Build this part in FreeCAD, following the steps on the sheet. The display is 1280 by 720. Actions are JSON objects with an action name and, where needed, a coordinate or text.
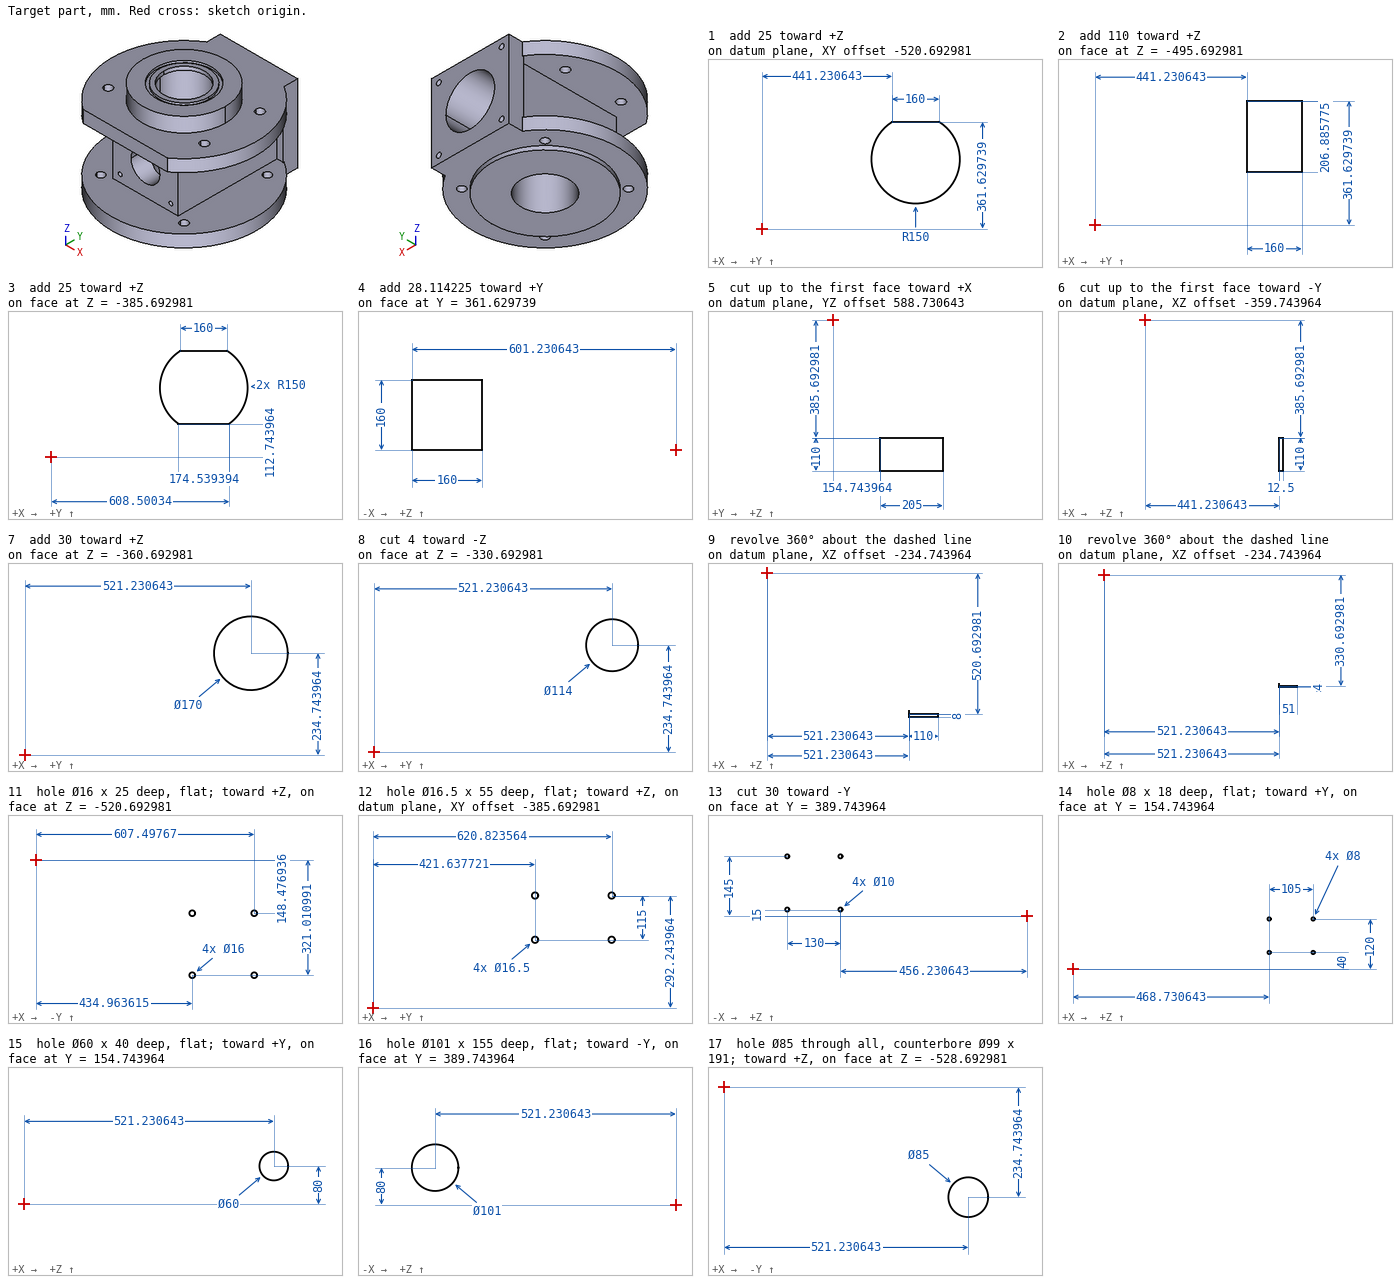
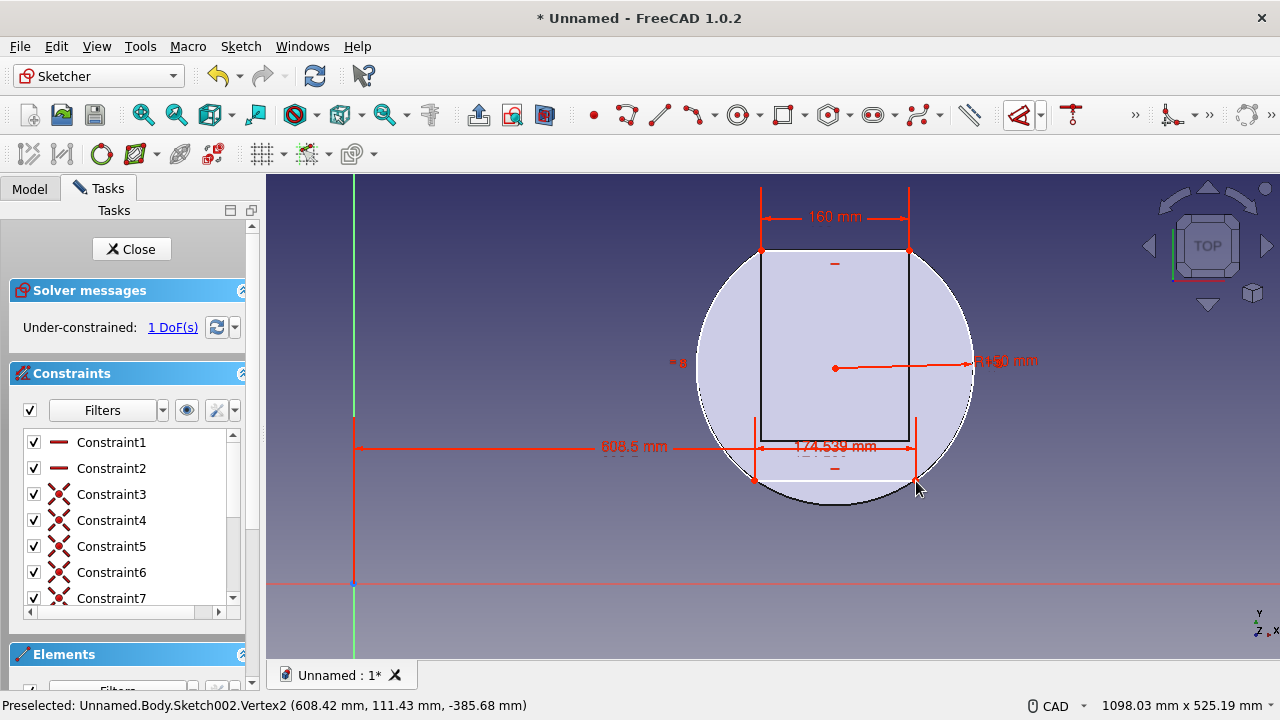
{"action": "left_click", "coordinate": [755, 481]}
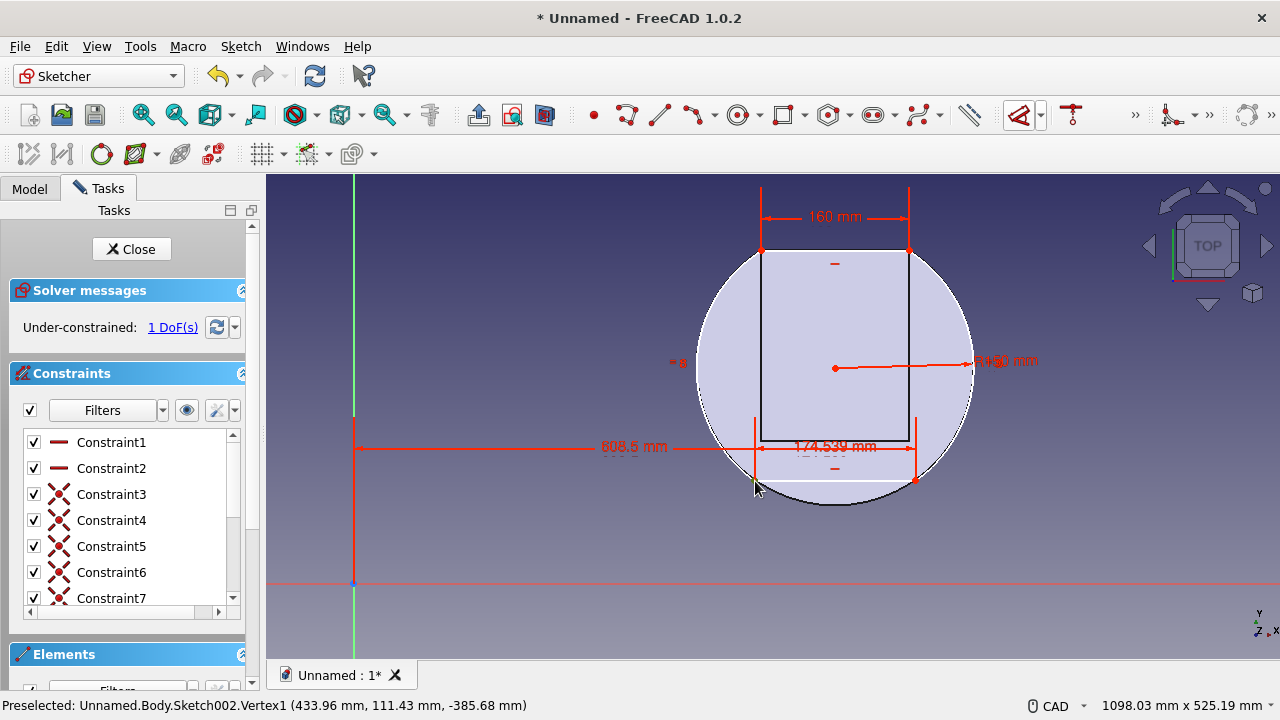
{"action": "left_click", "coordinate": [1040, 116]}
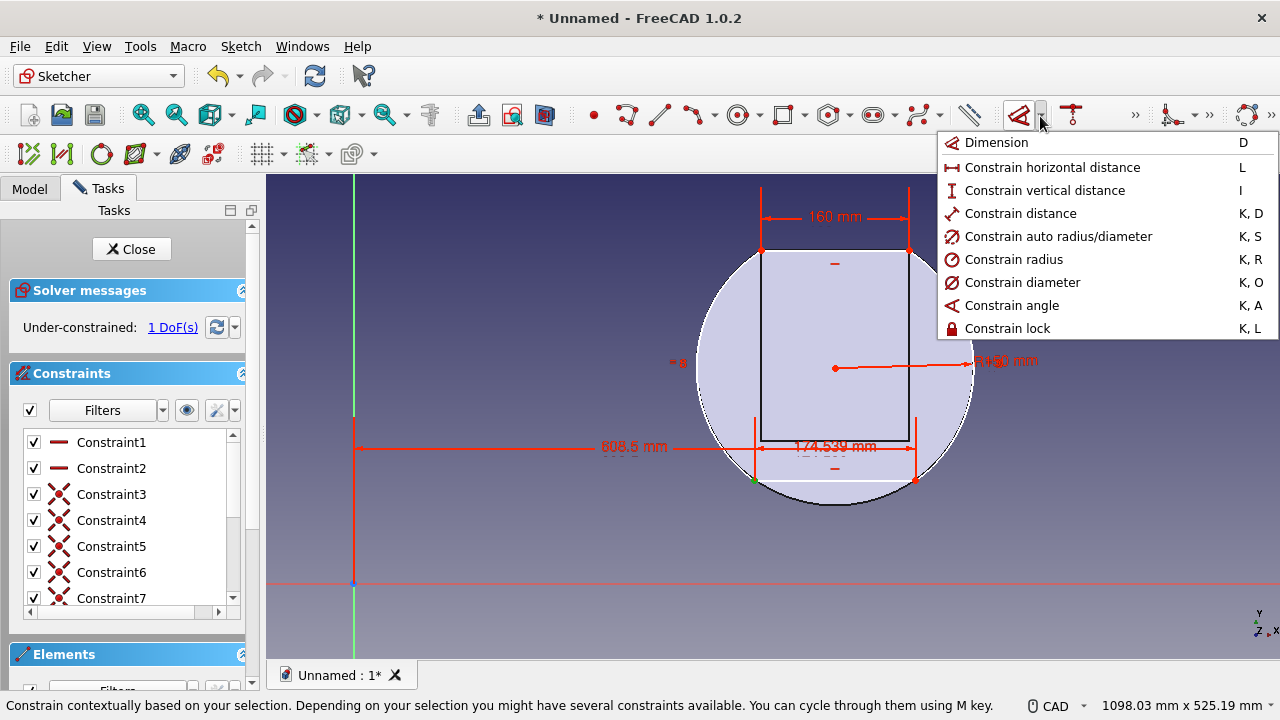
{"action": "left_click", "coordinate": [1108, 190]}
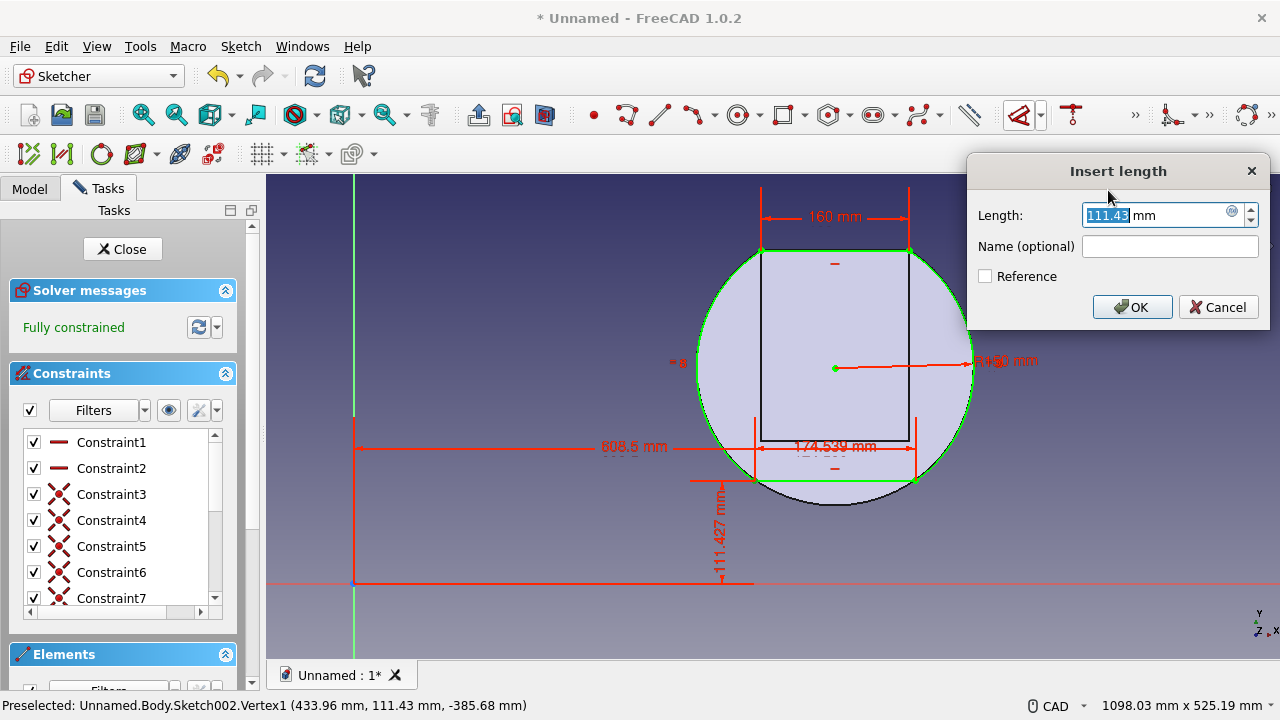
{"action": "type", "text": "112.743964"}
{"action": "key", "text": "Return"}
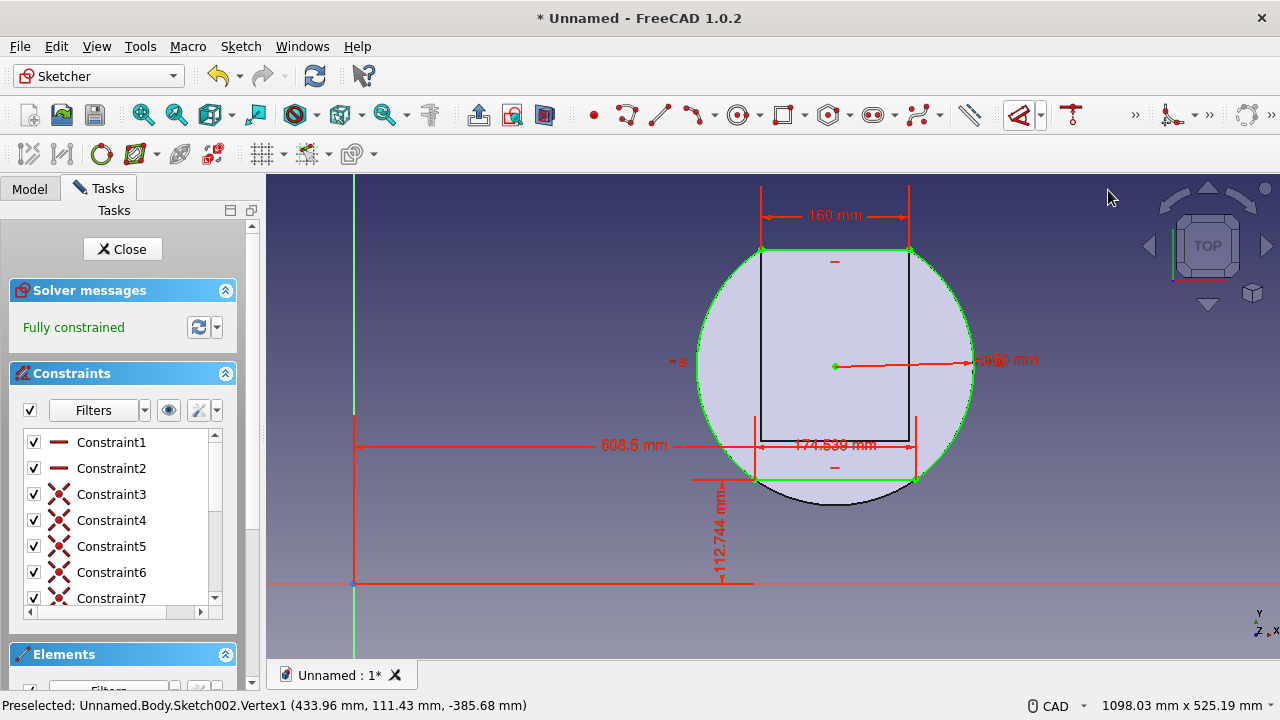
{"action": "left_click", "coordinate": [123, 249]}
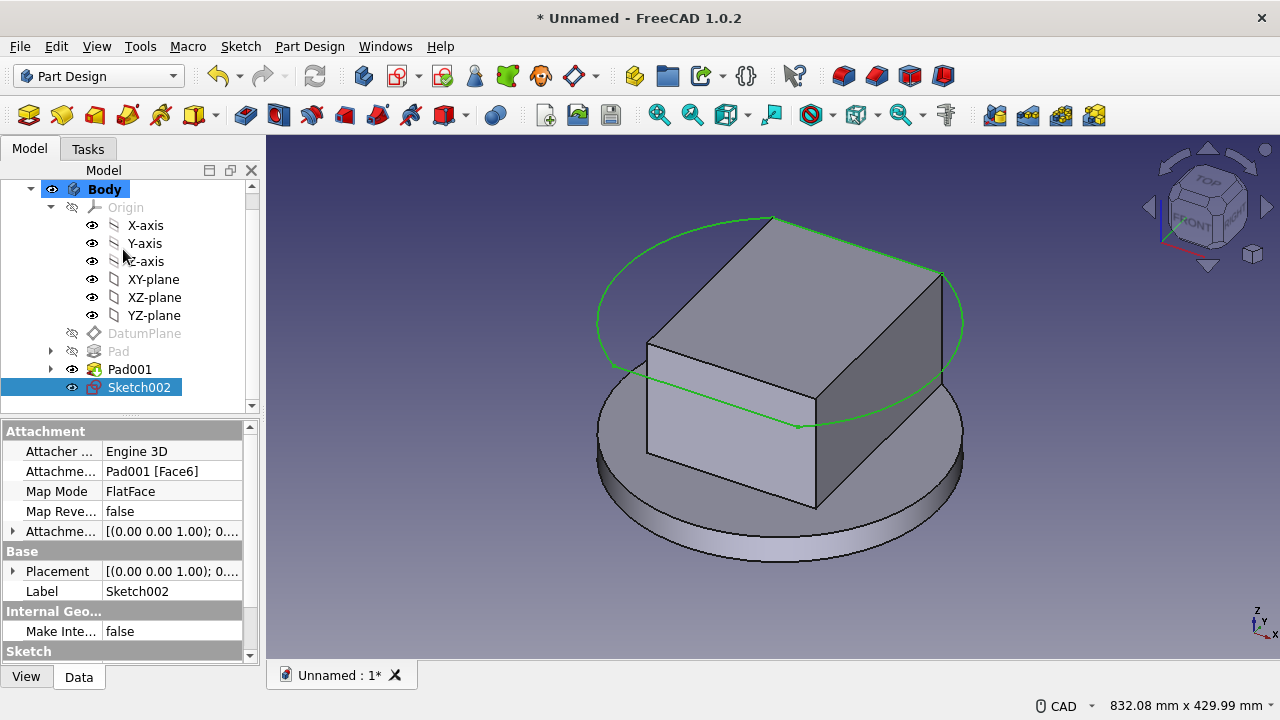
{"action": "left_click", "coordinate": [29, 116]}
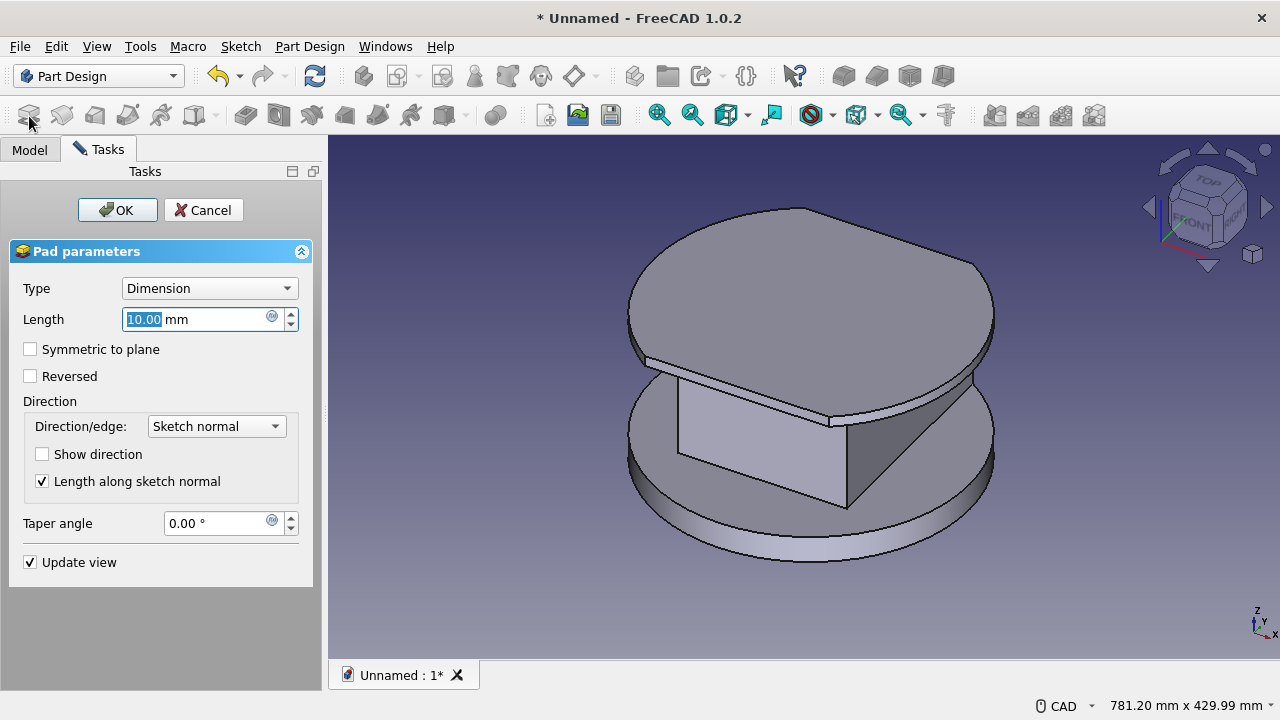
{"action": "type", "text": "25"}
{"action": "key", "text": "Tab"}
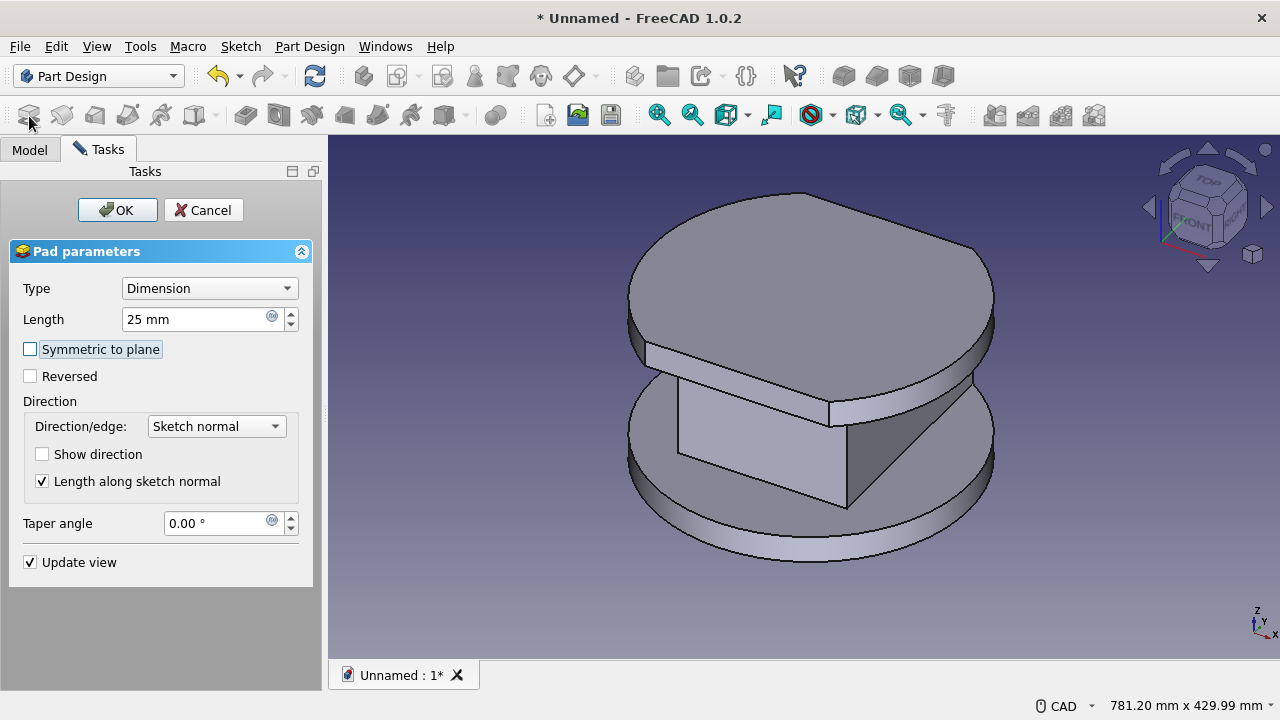
{"action": "left_click", "coordinate": [118, 210]}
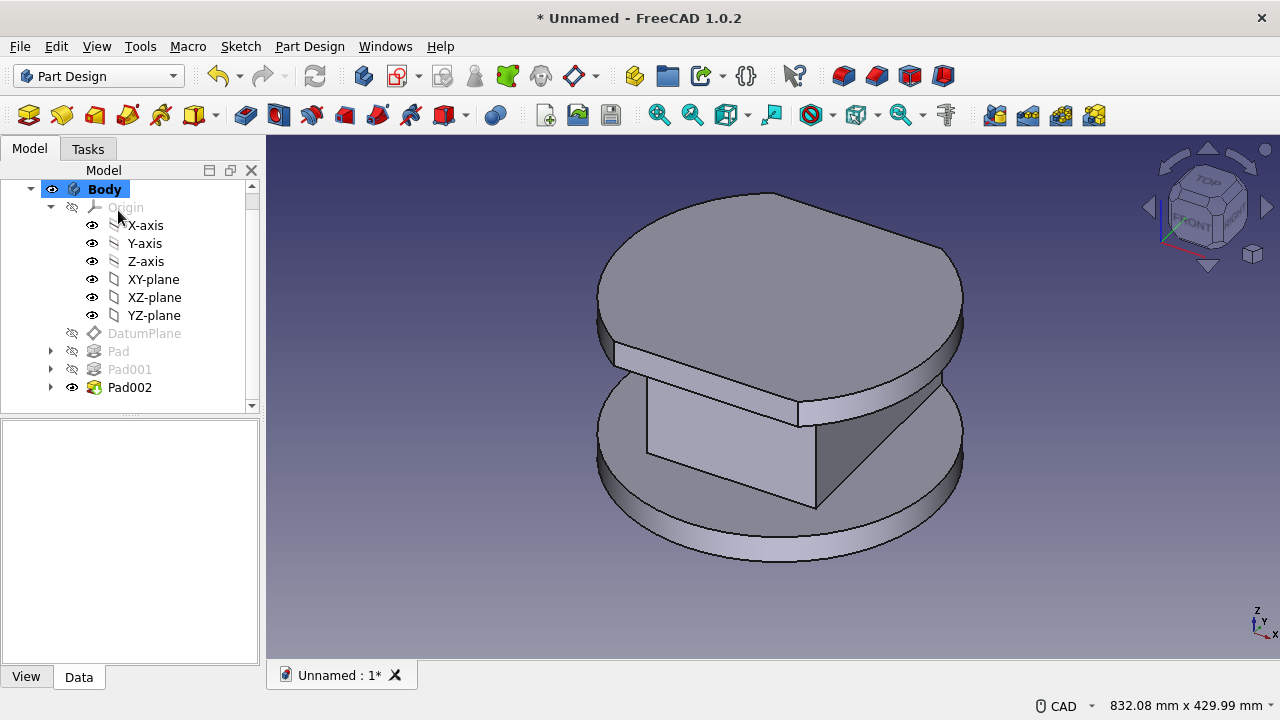
{"action": "key", "text": "4"}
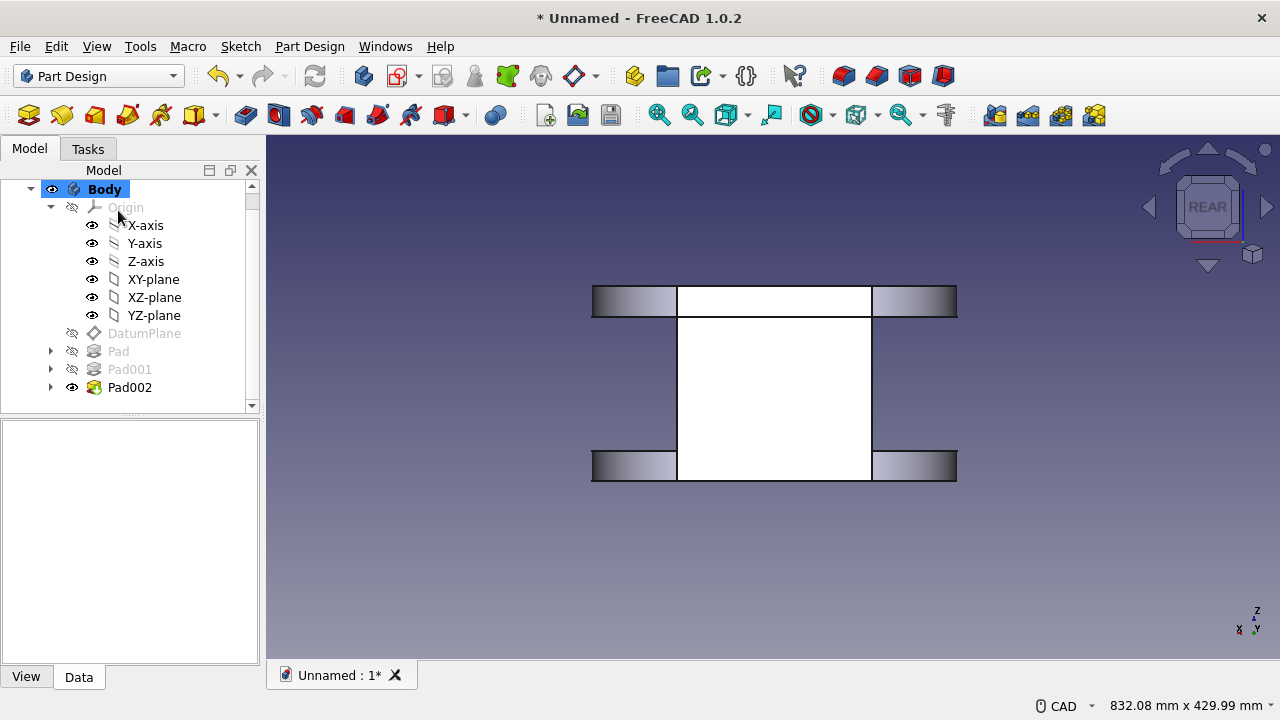
{"action": "left_click", "coordinate": [660, 116]}